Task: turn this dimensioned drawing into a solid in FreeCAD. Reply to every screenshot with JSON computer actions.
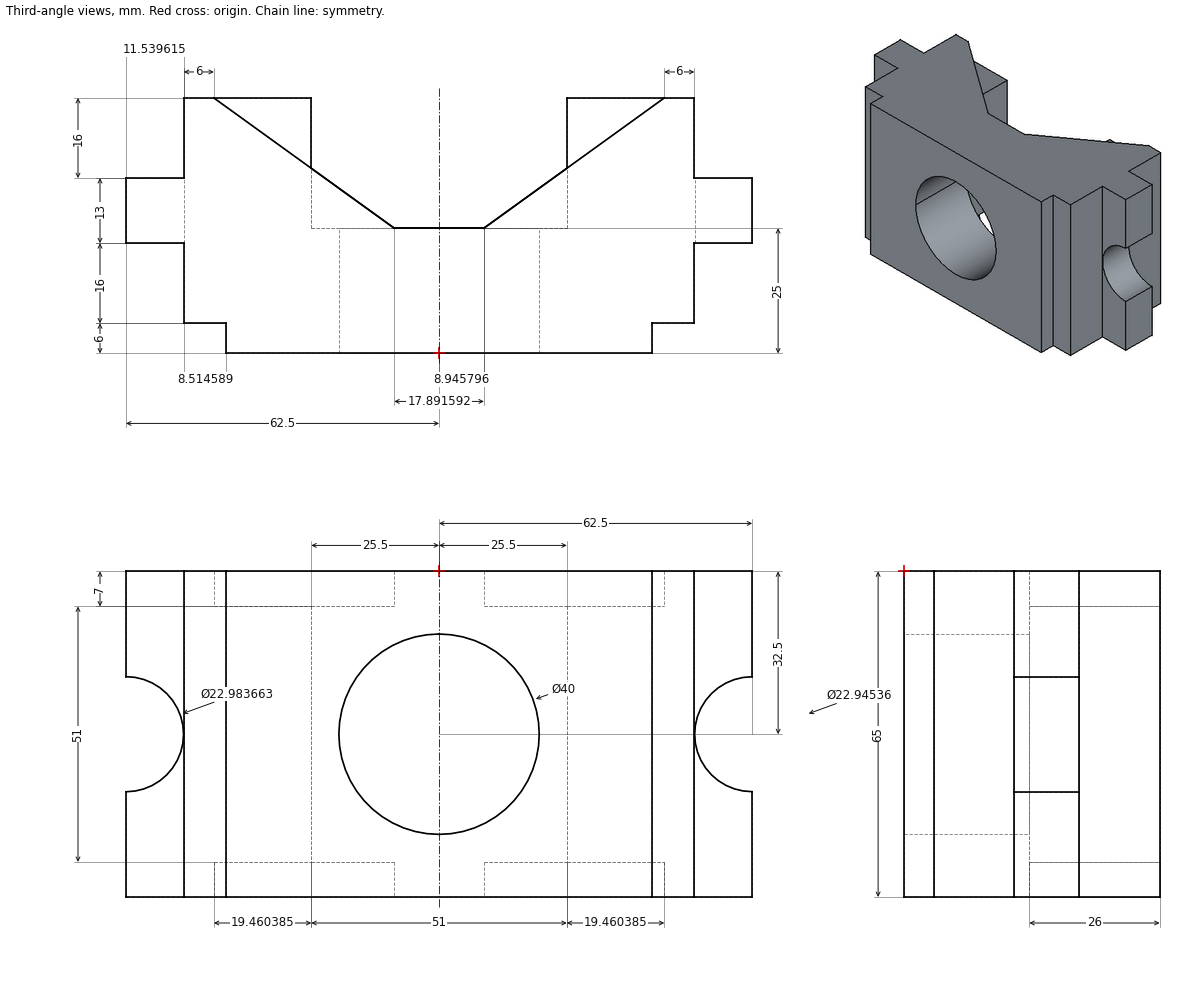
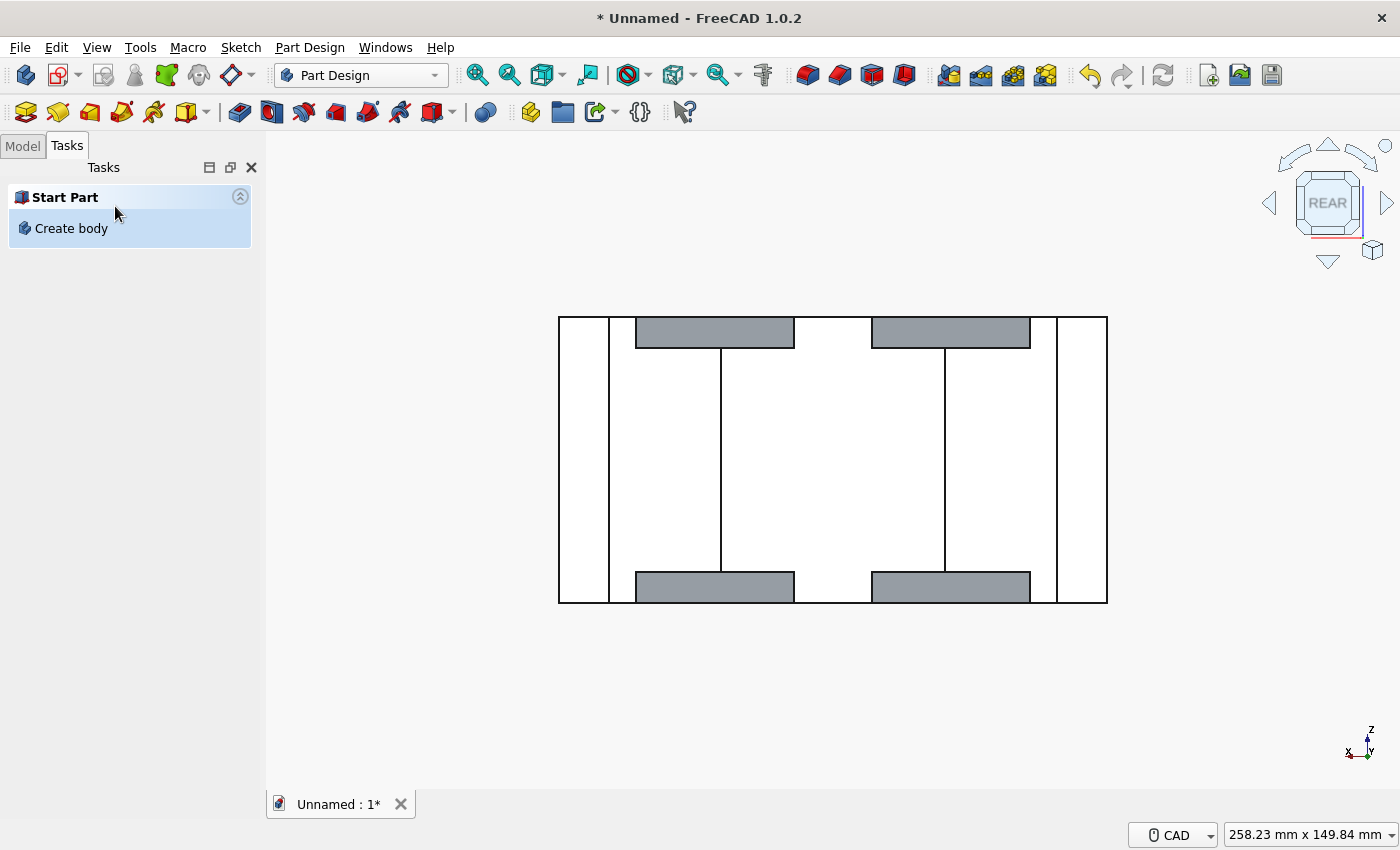
{"action": "left_click", "coordinate": [833, 459]}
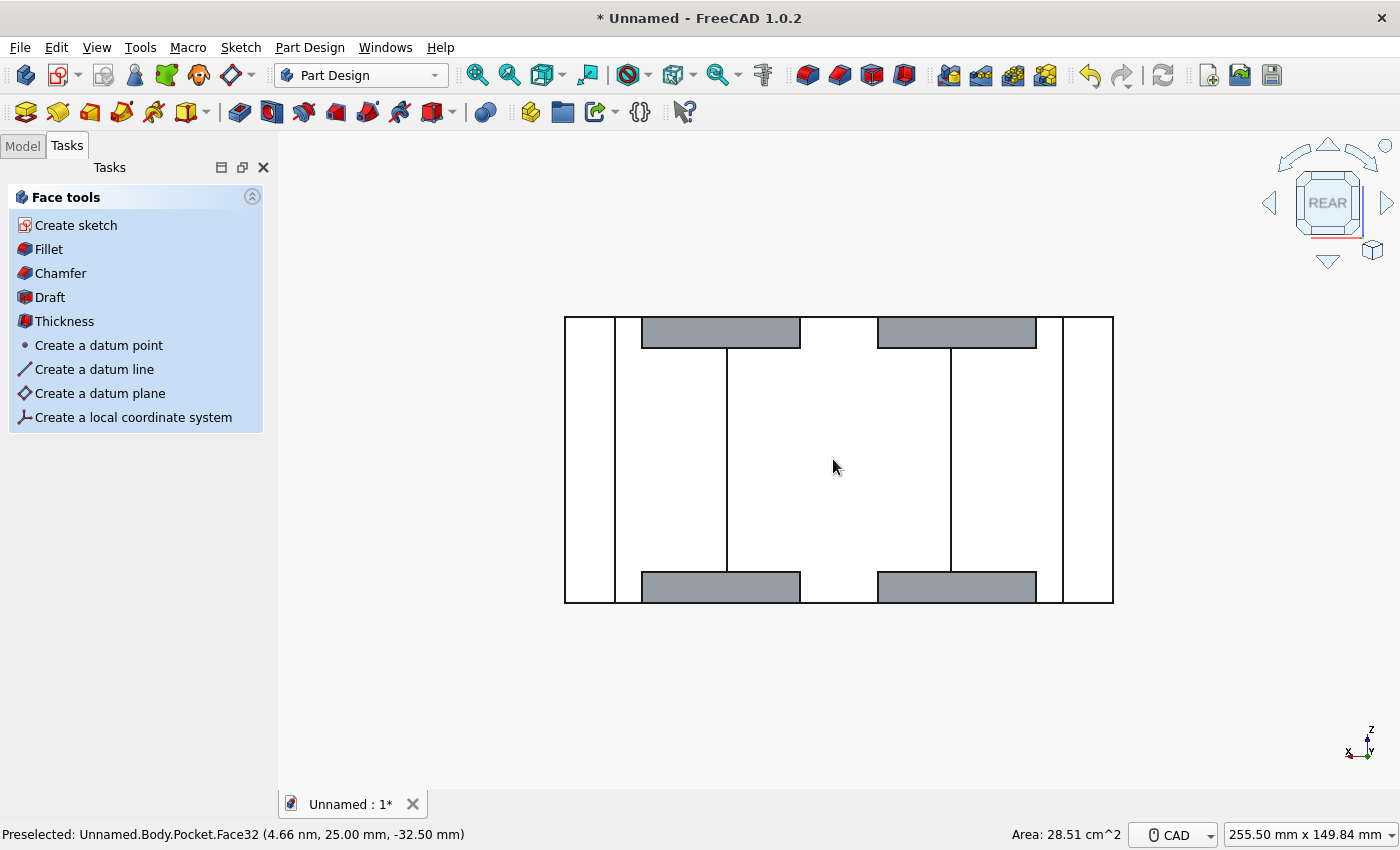
{"action": "left_click", "coordinate": [58, 76]}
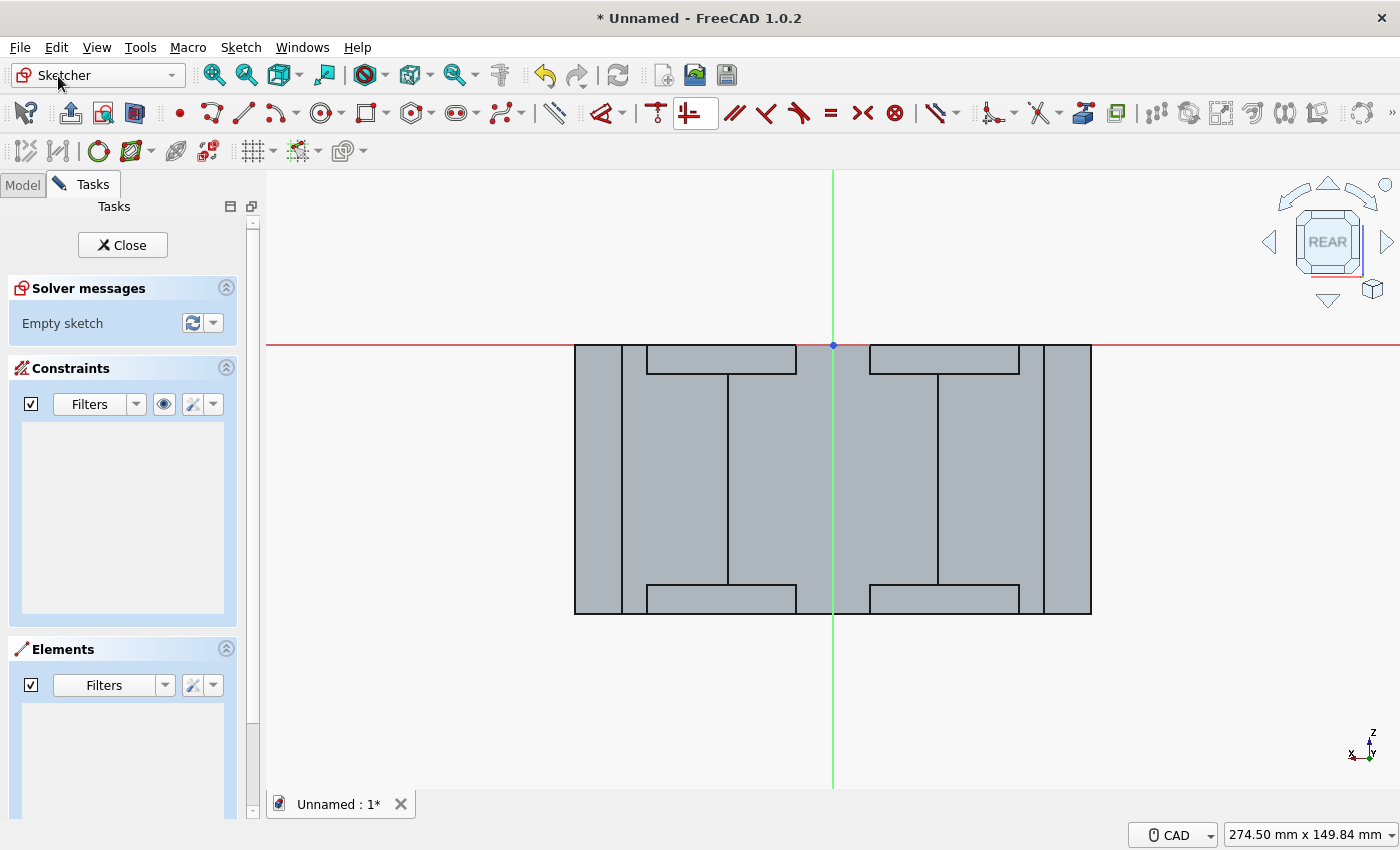
{"action": "left_click", "coordinate": [136, 114]}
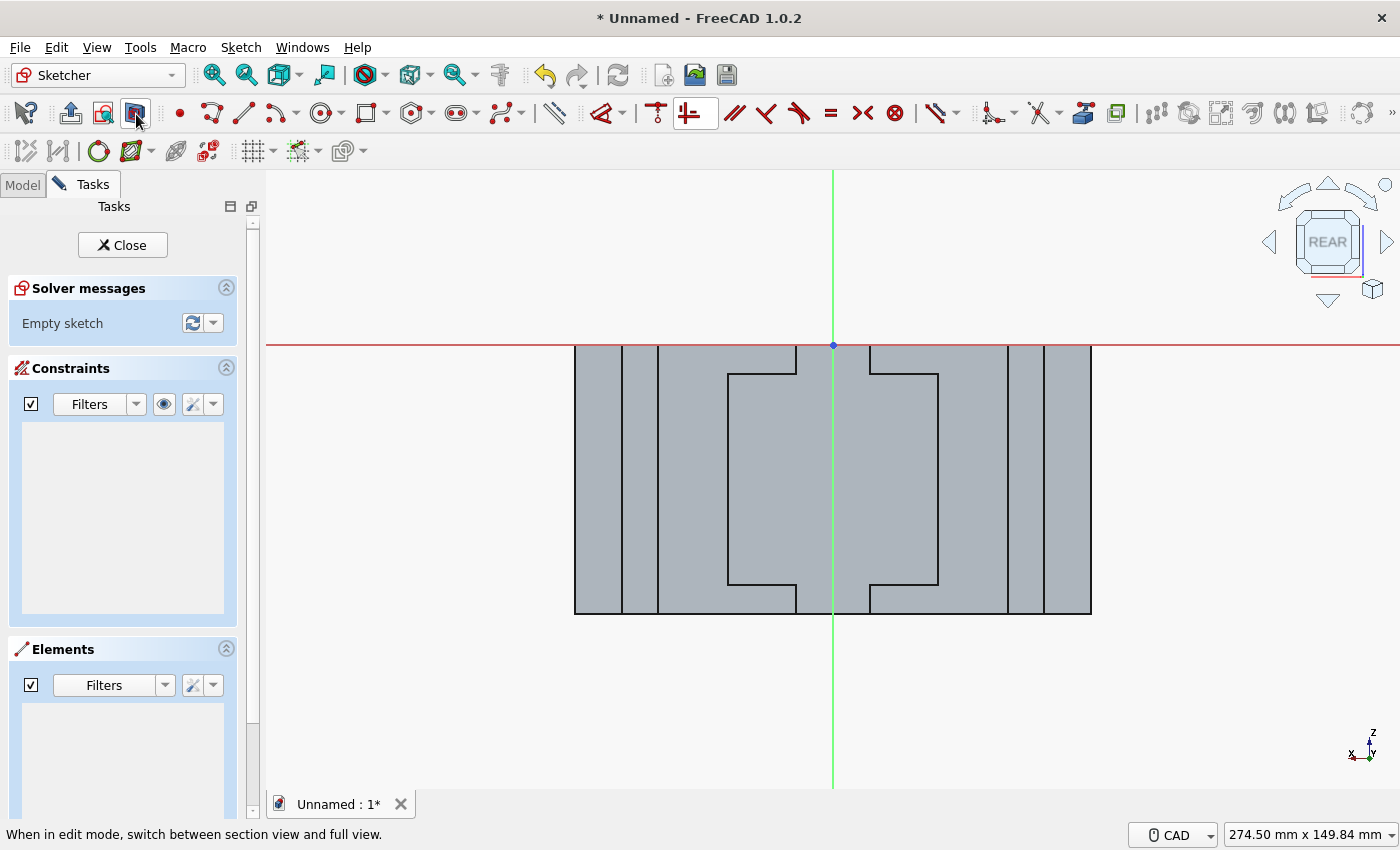
{"action": "scroll", "coordinate": [916, 422], "scroll_direction": "up", "scroll_amount": 3}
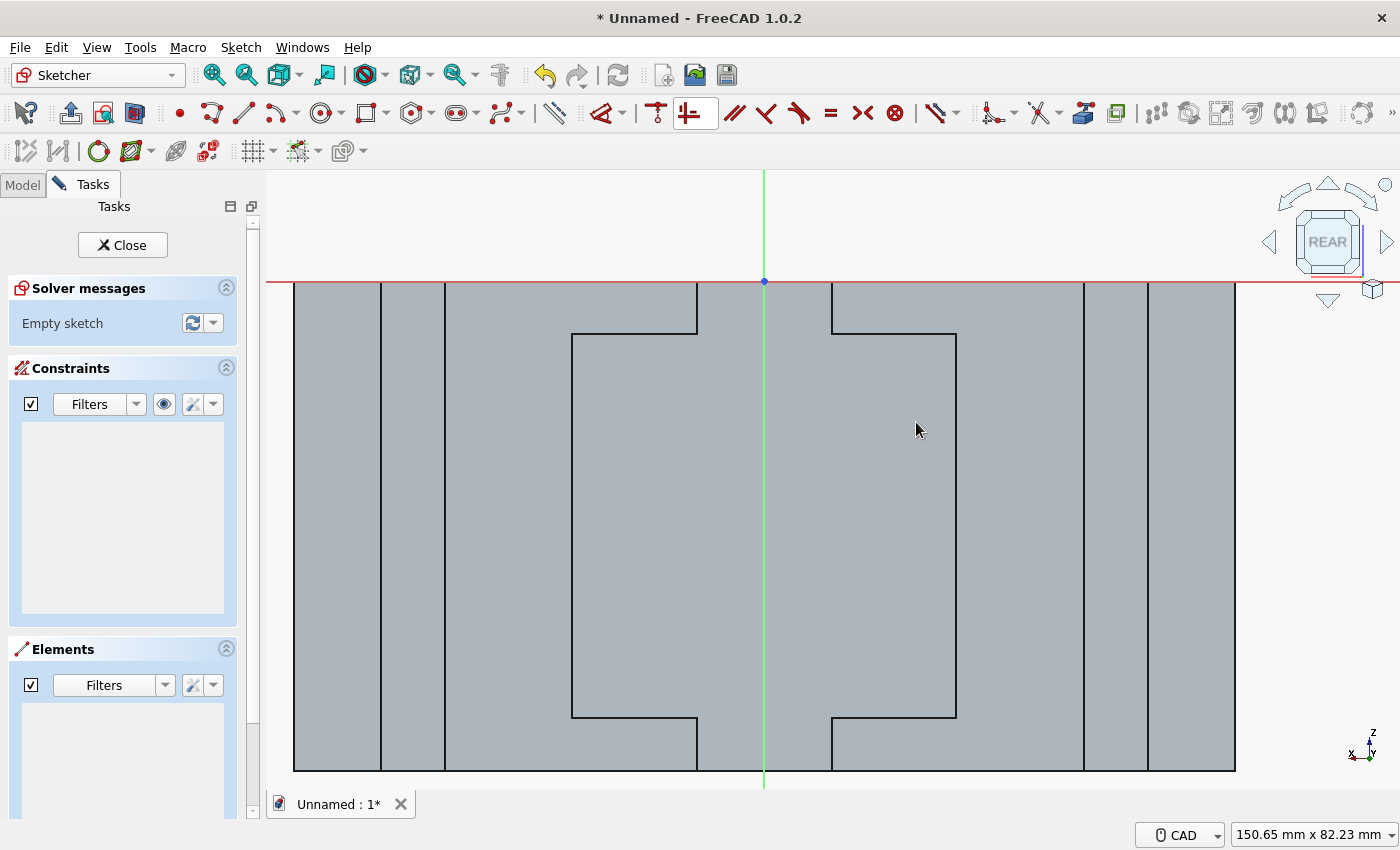
{"action": "left_click", "coordinate": [322, 114]}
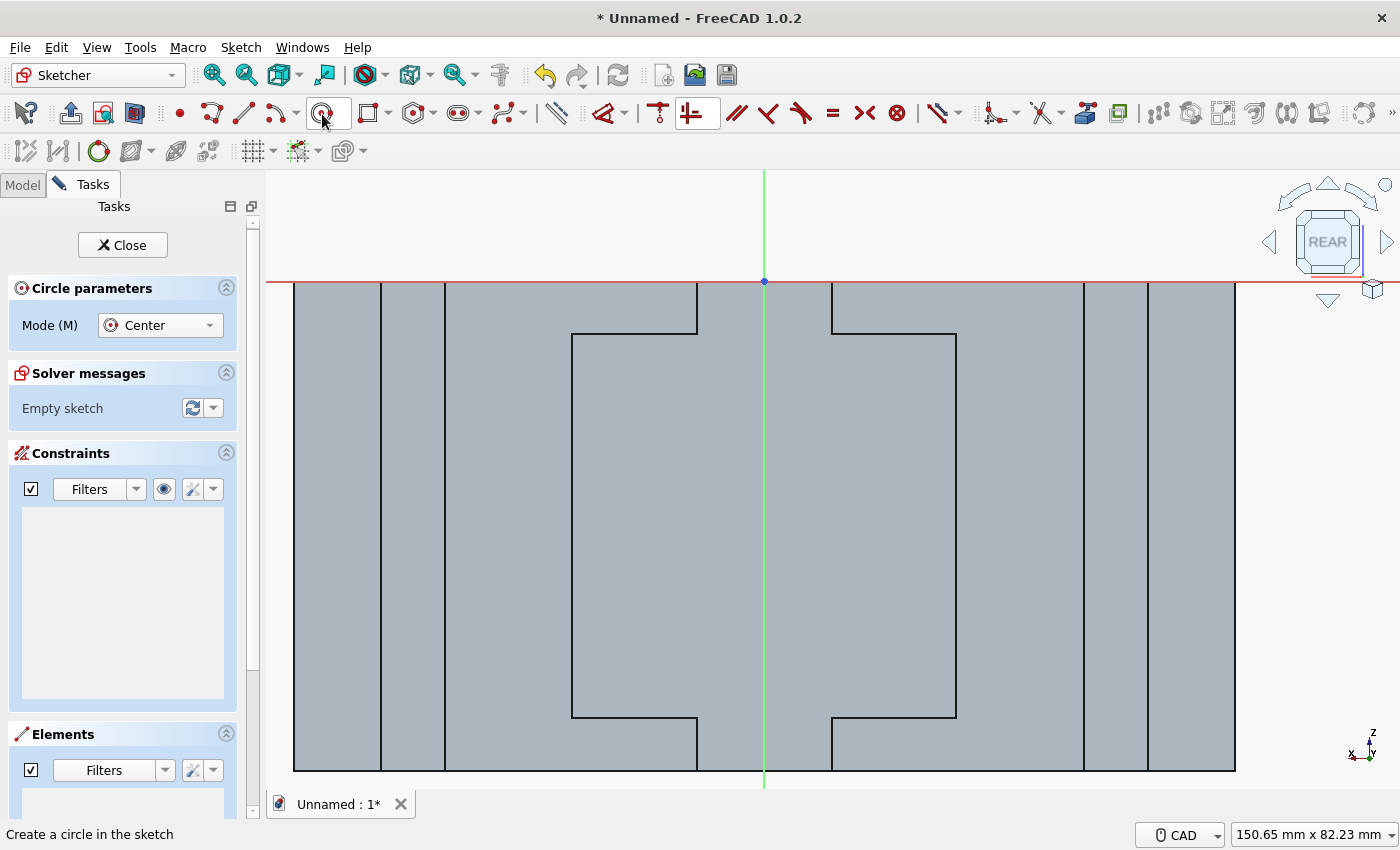
{"action": "left_click", "coordinate": [764, 526]}
{"action": "mouse_move", "coordinate": [871, 420]}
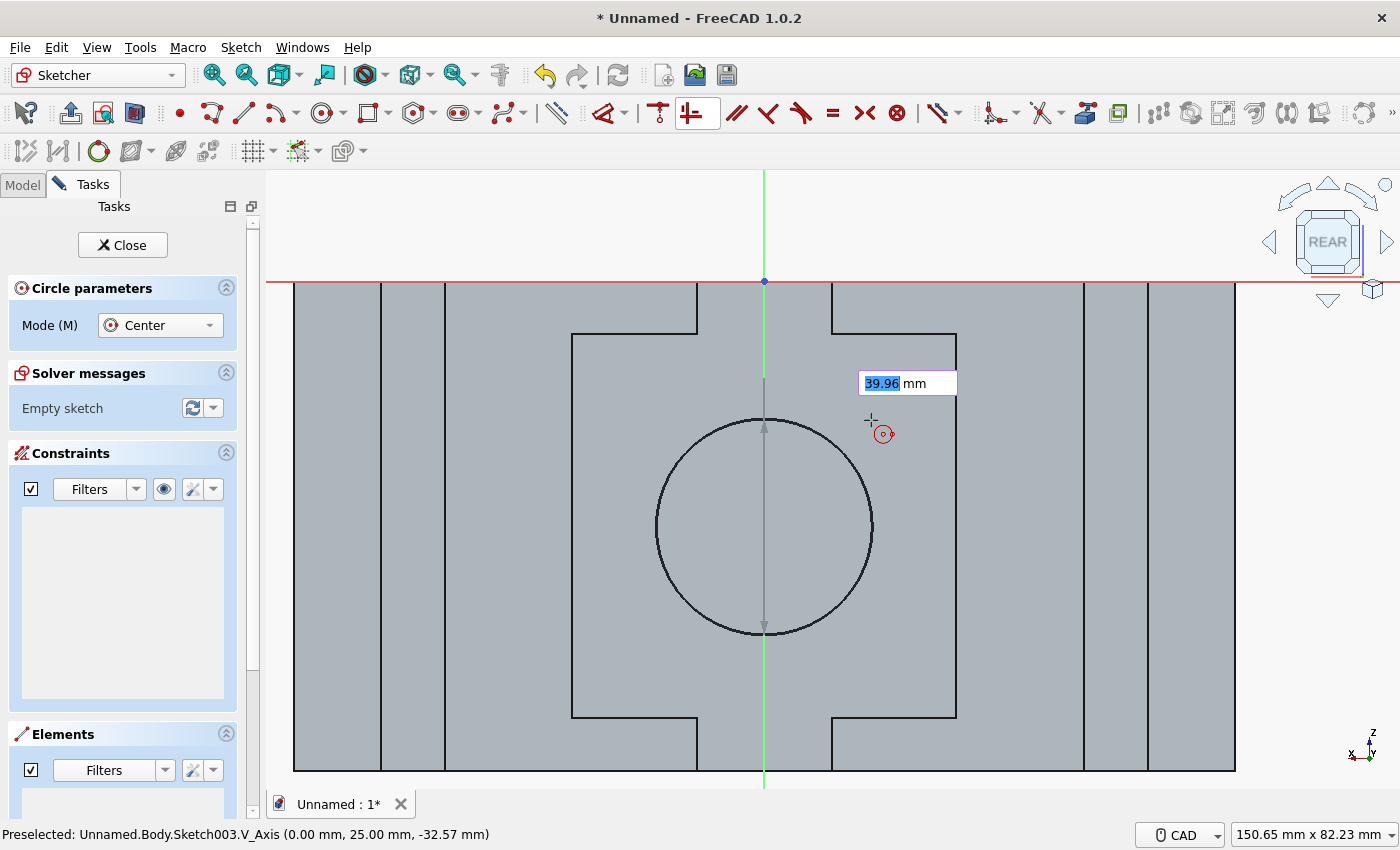
{"action": "type", "text": "40"}
{"action": "key", "text": "Return"}
{"action": "key", "text": "Escape"}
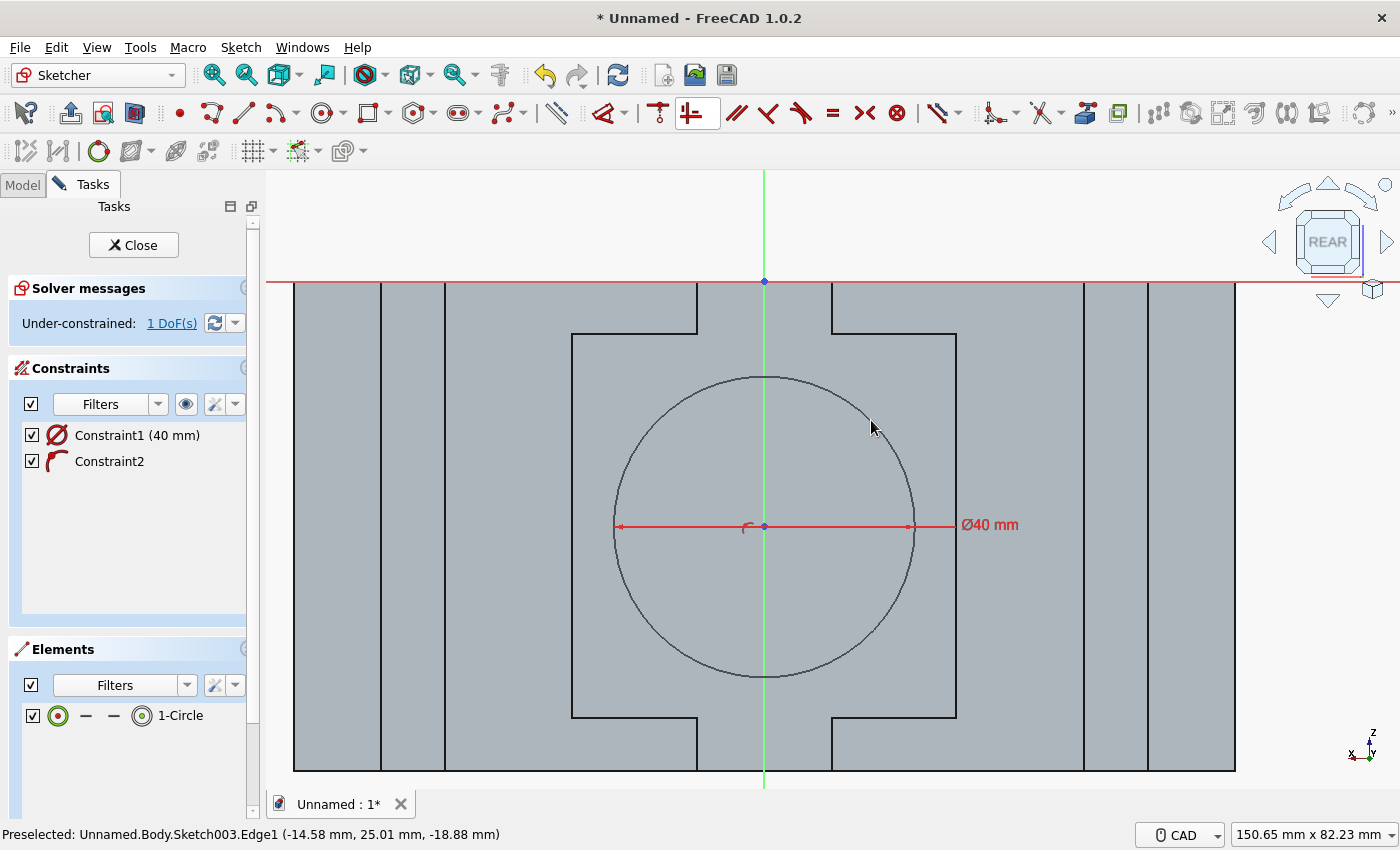
{"action": "left_click", "coordinate": [604, 114]}